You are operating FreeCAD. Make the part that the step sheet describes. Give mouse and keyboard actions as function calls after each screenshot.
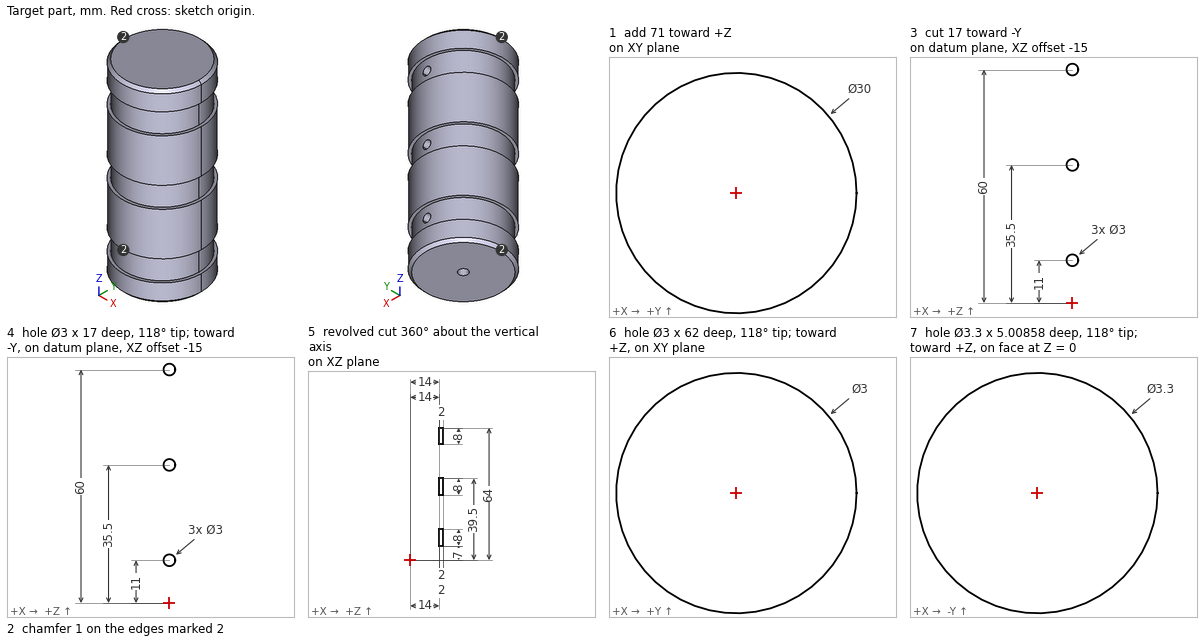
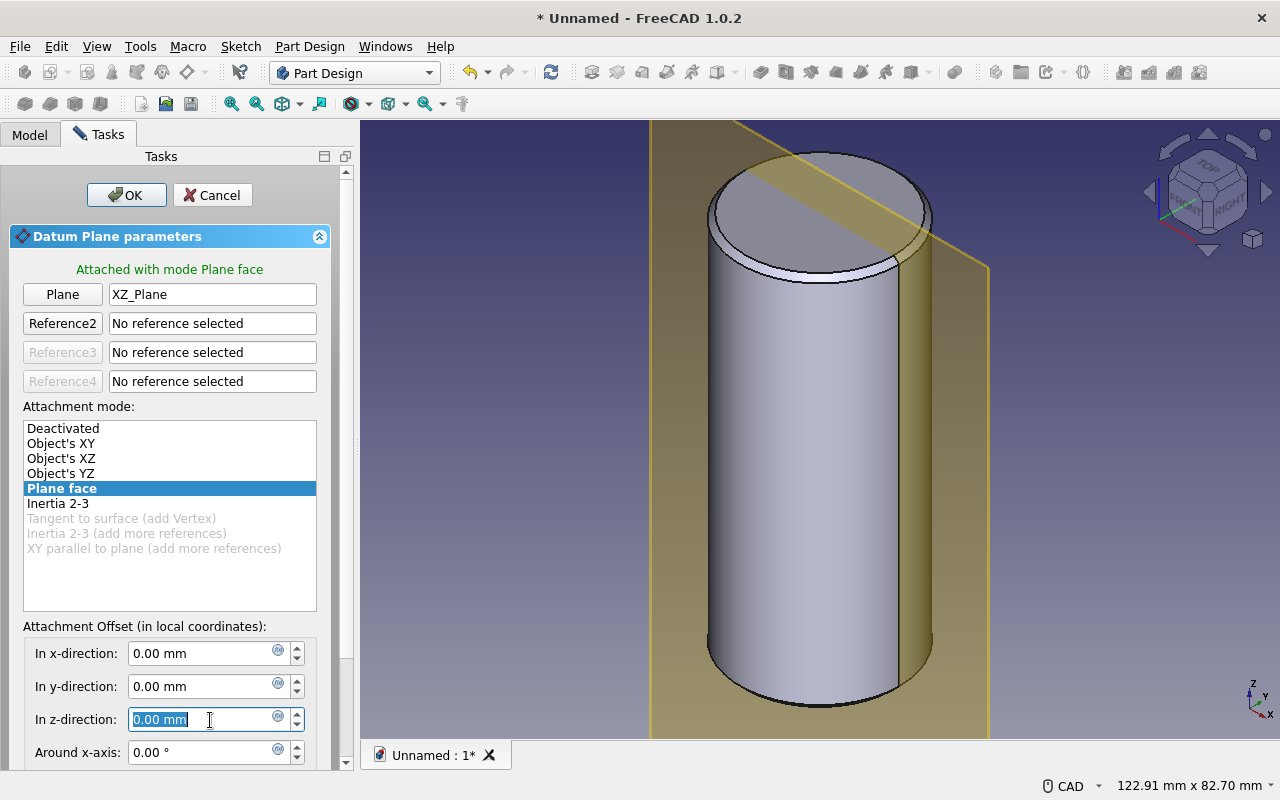
text(-15)
key(Tab)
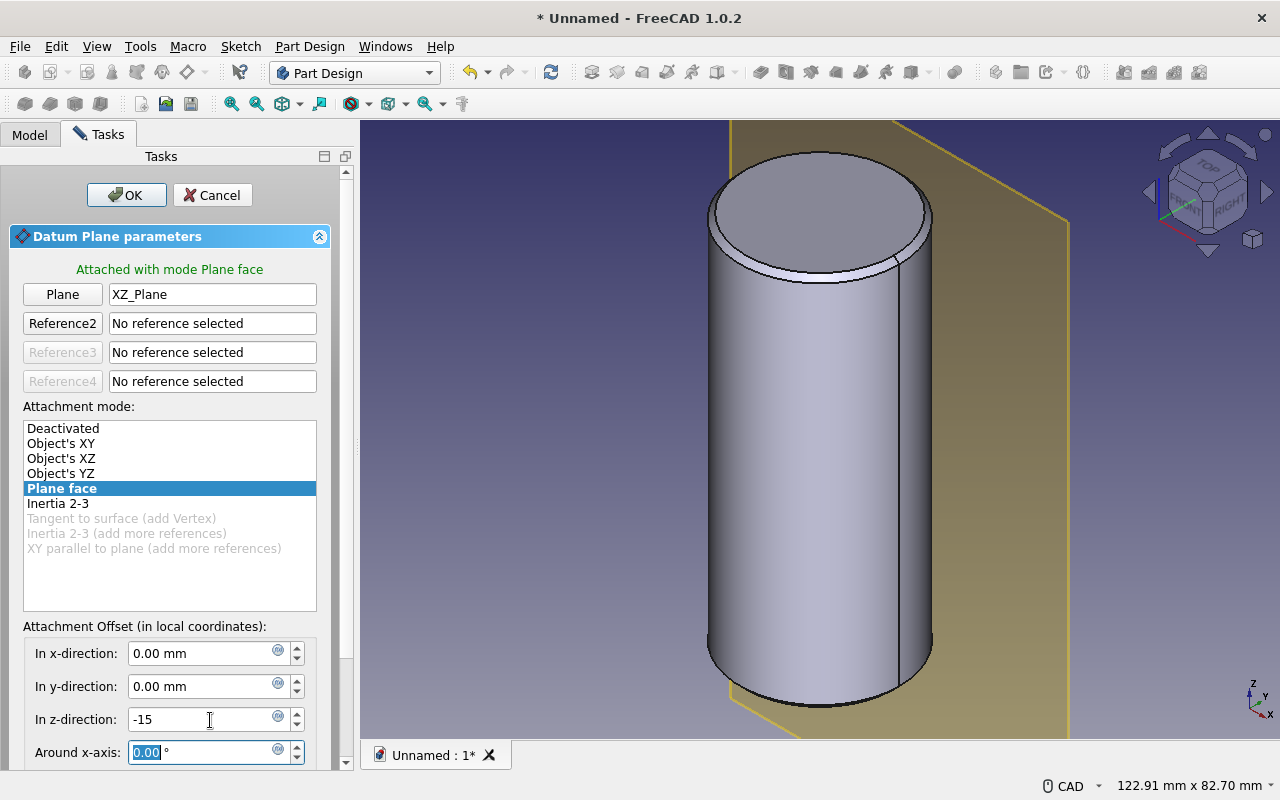
click(127, 195)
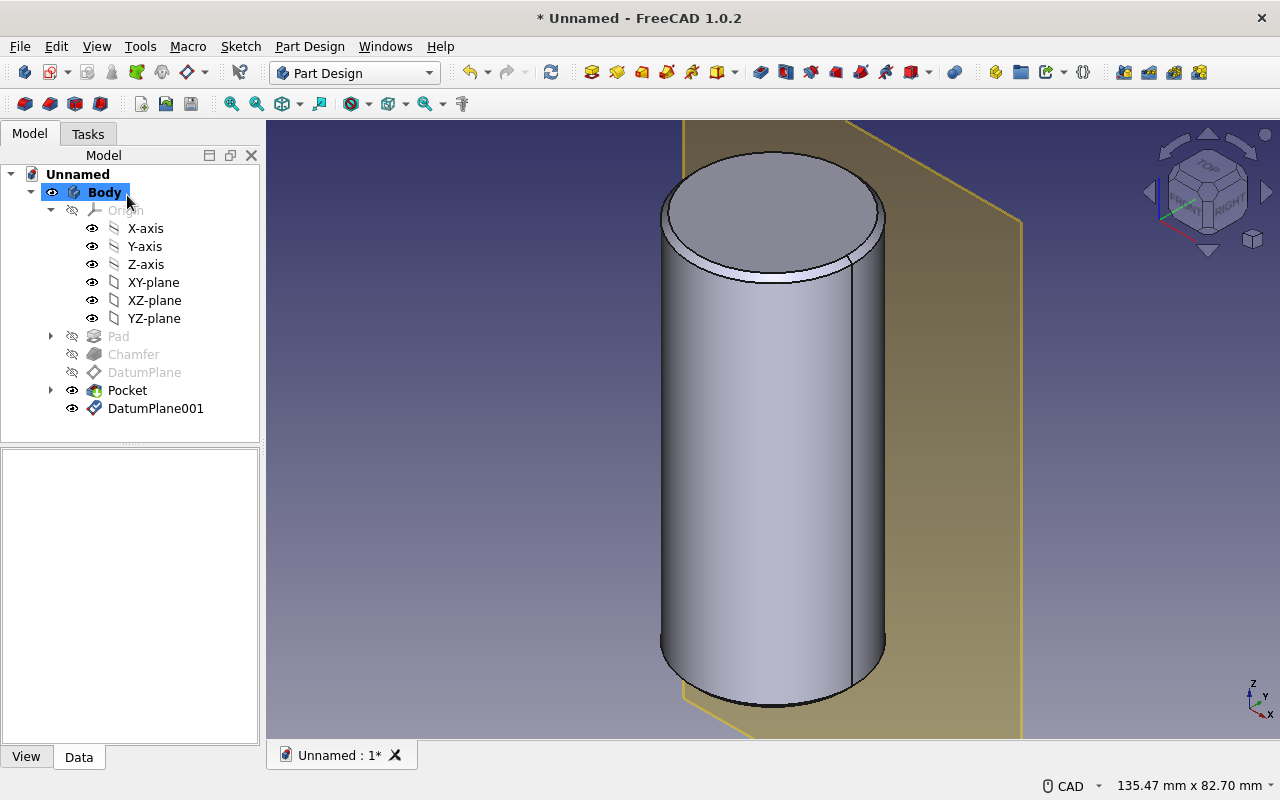
click(117, 408)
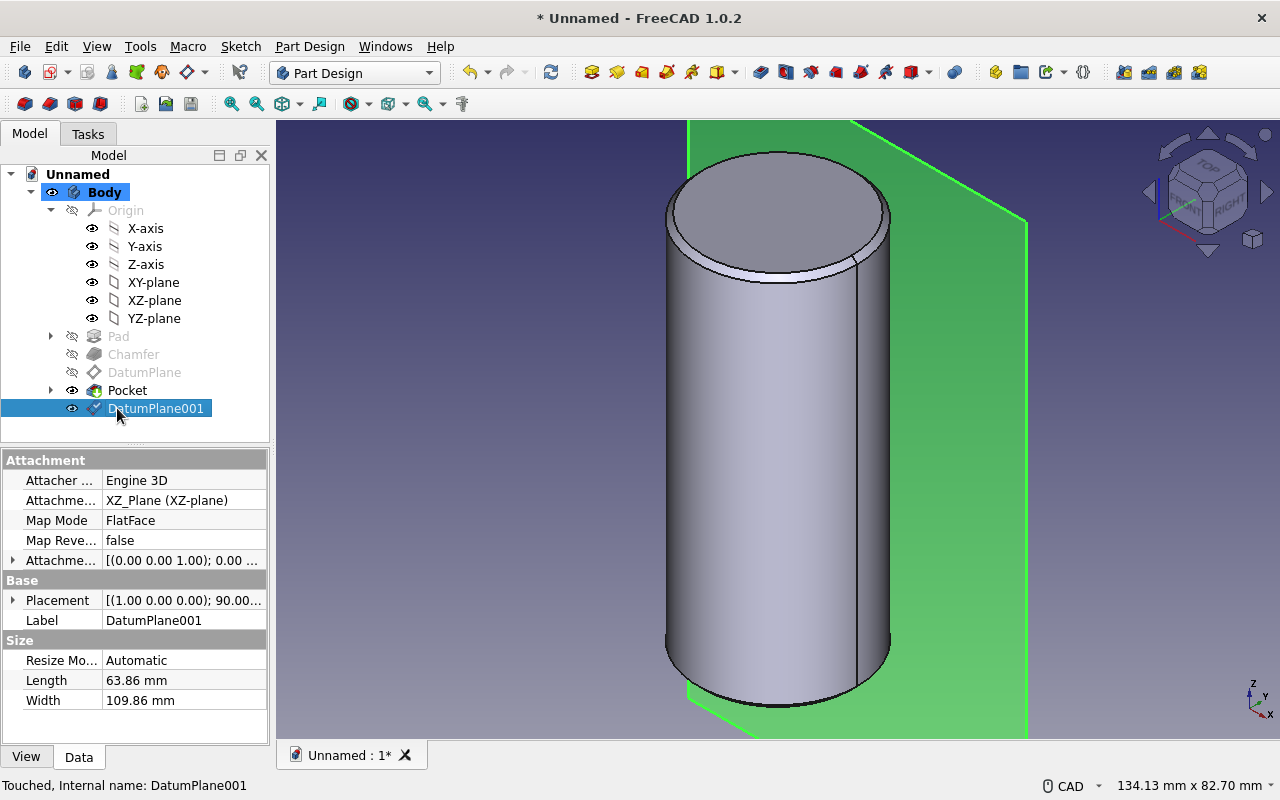
click(50, 72)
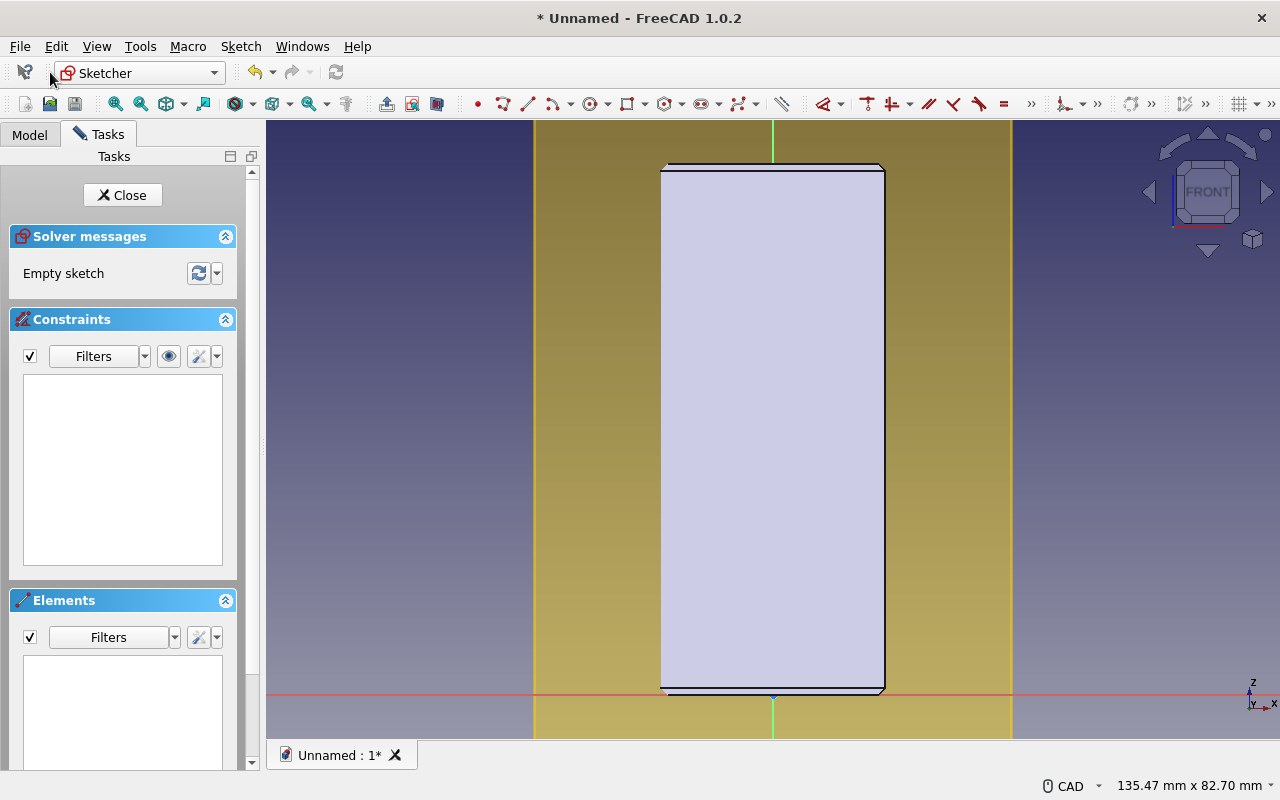
click(437, 104)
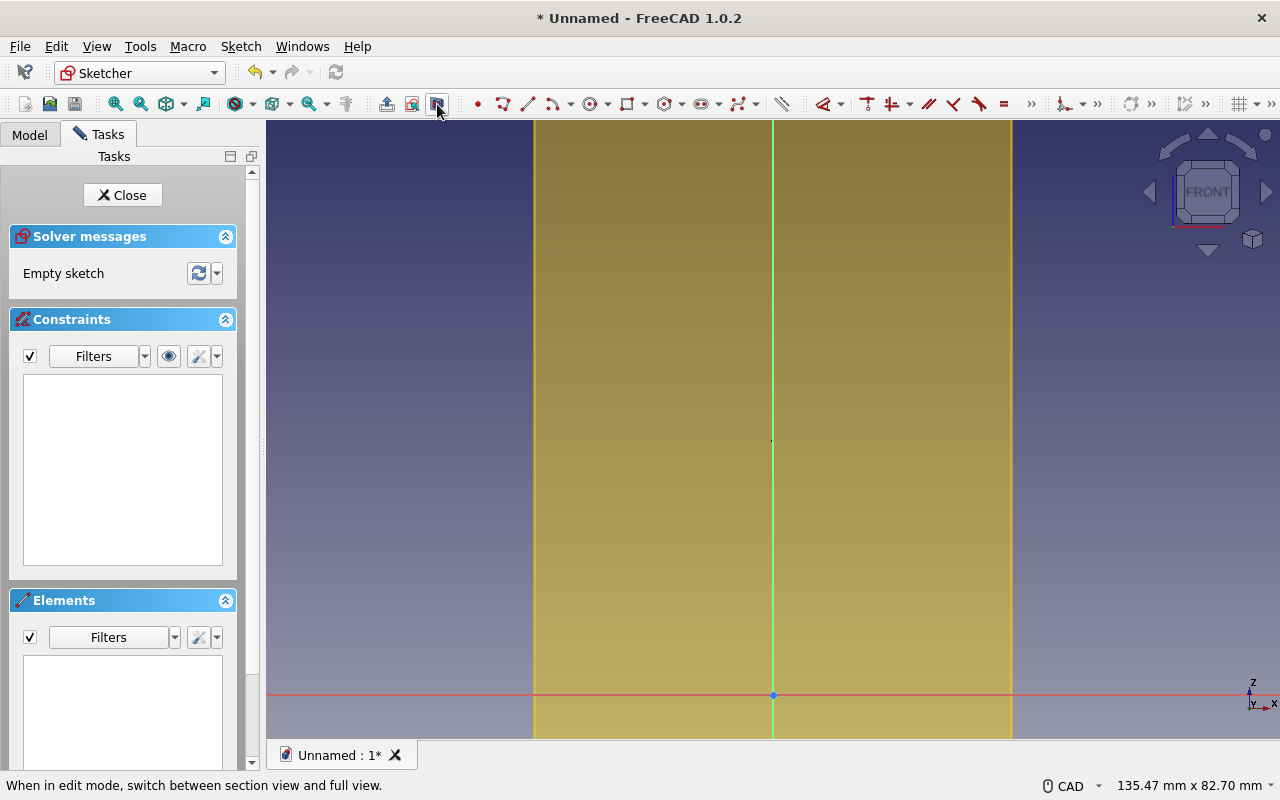
scroll(395, 269, down, 1)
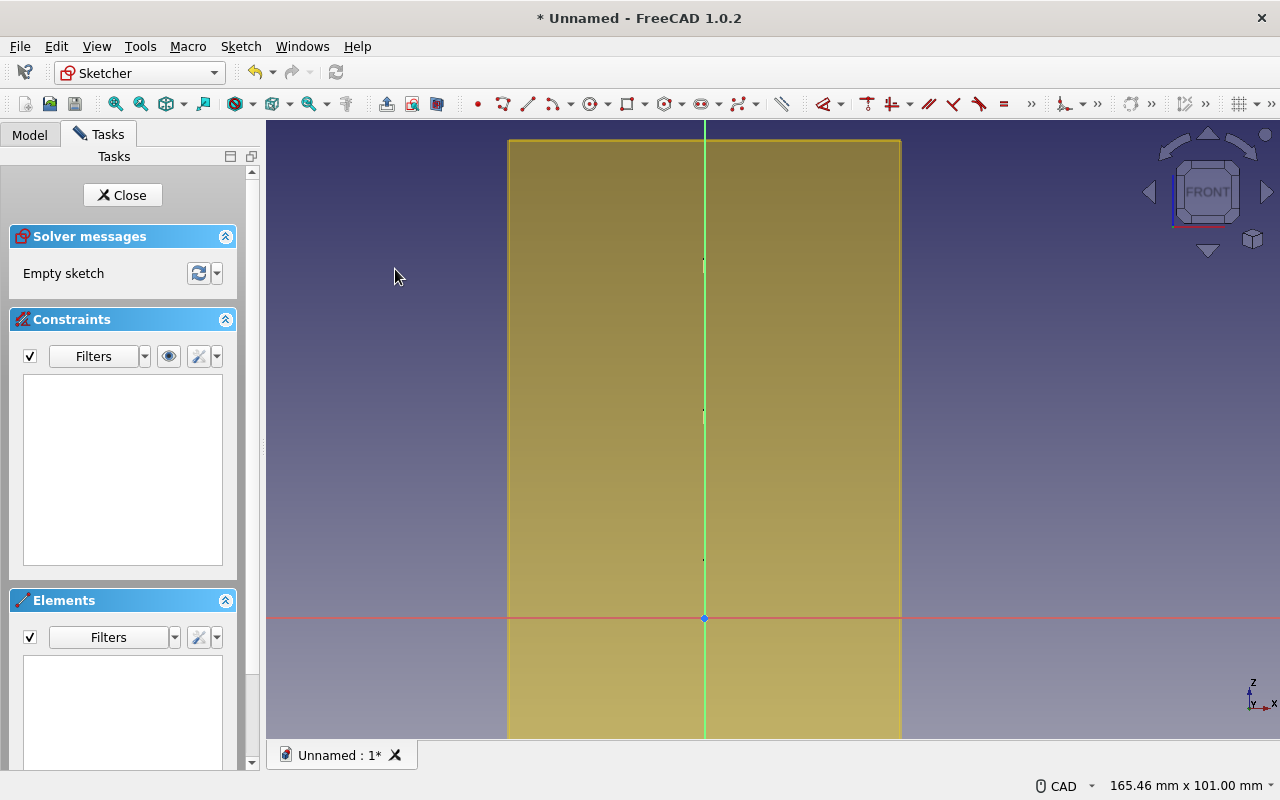
click(590, 104)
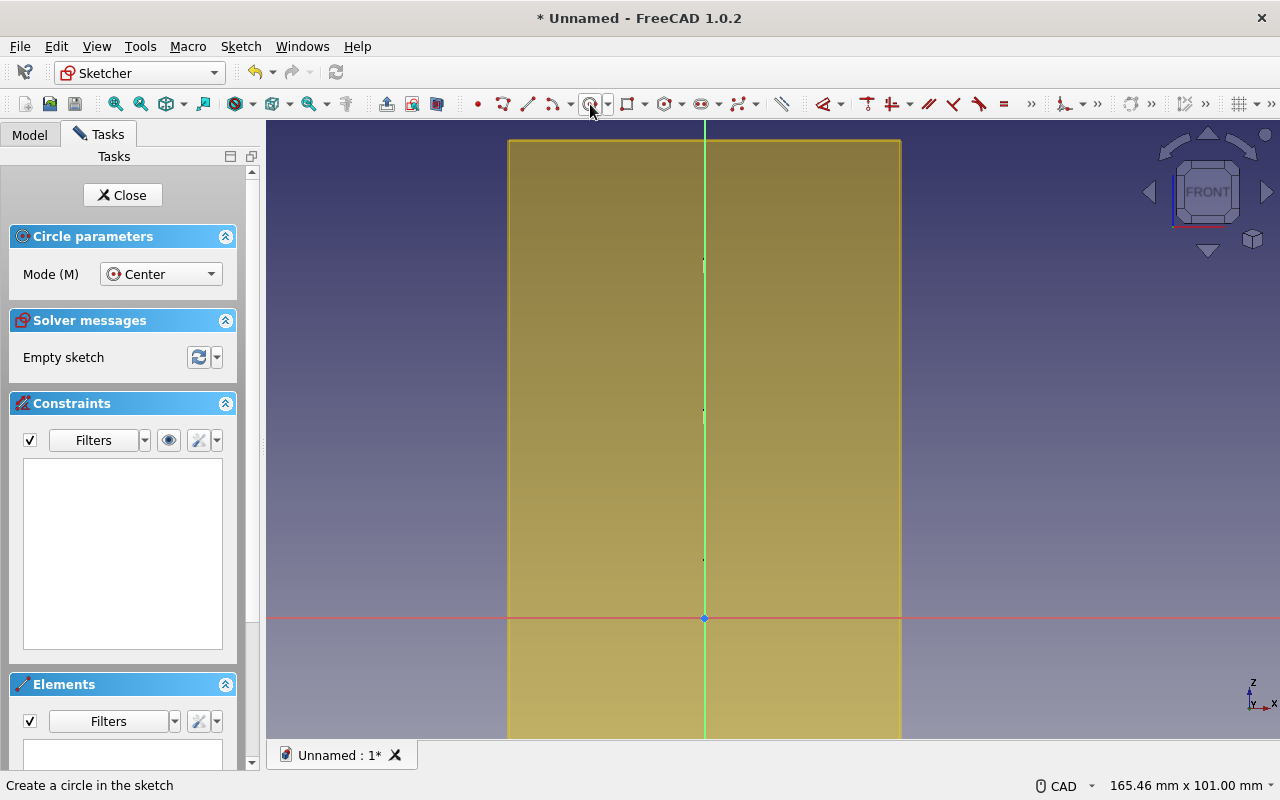
scroll(705, 551, up, 5)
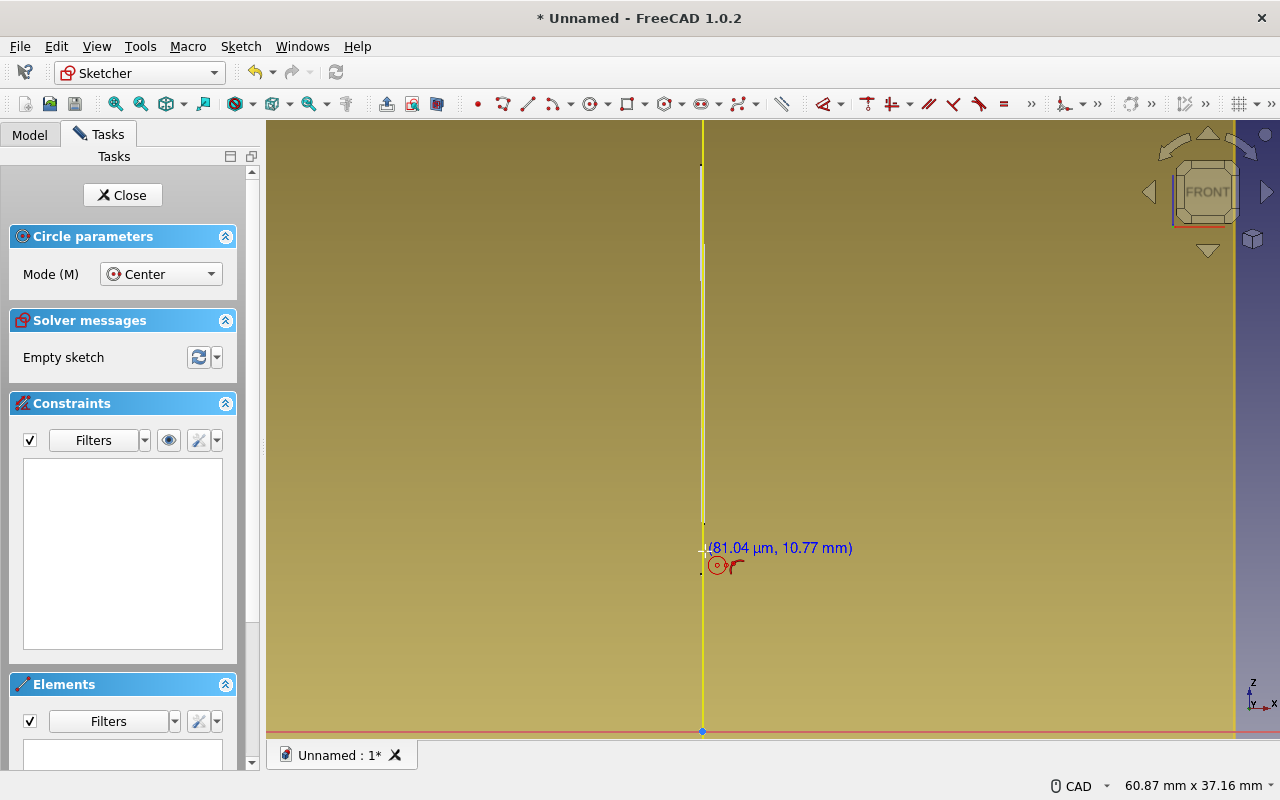
click(703, 549)
move(721, 531)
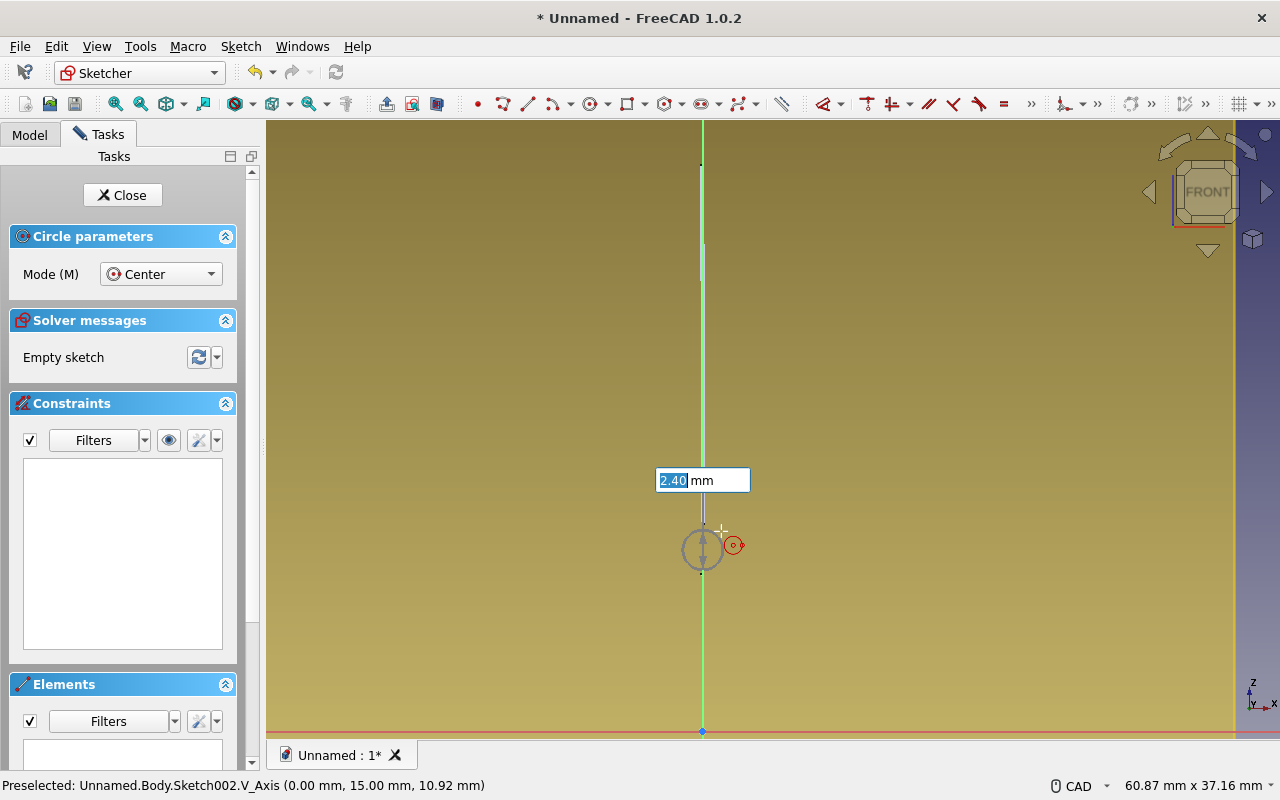
text(3)
key(Return)